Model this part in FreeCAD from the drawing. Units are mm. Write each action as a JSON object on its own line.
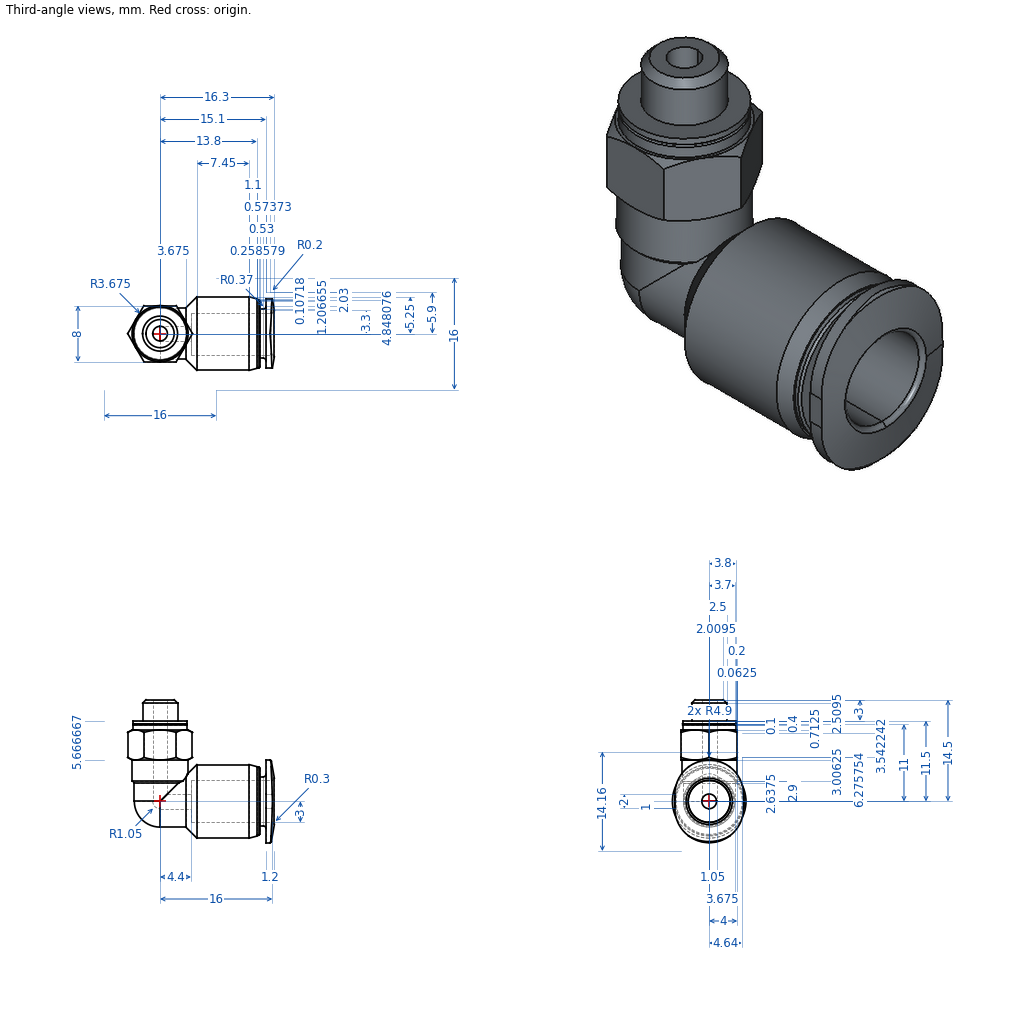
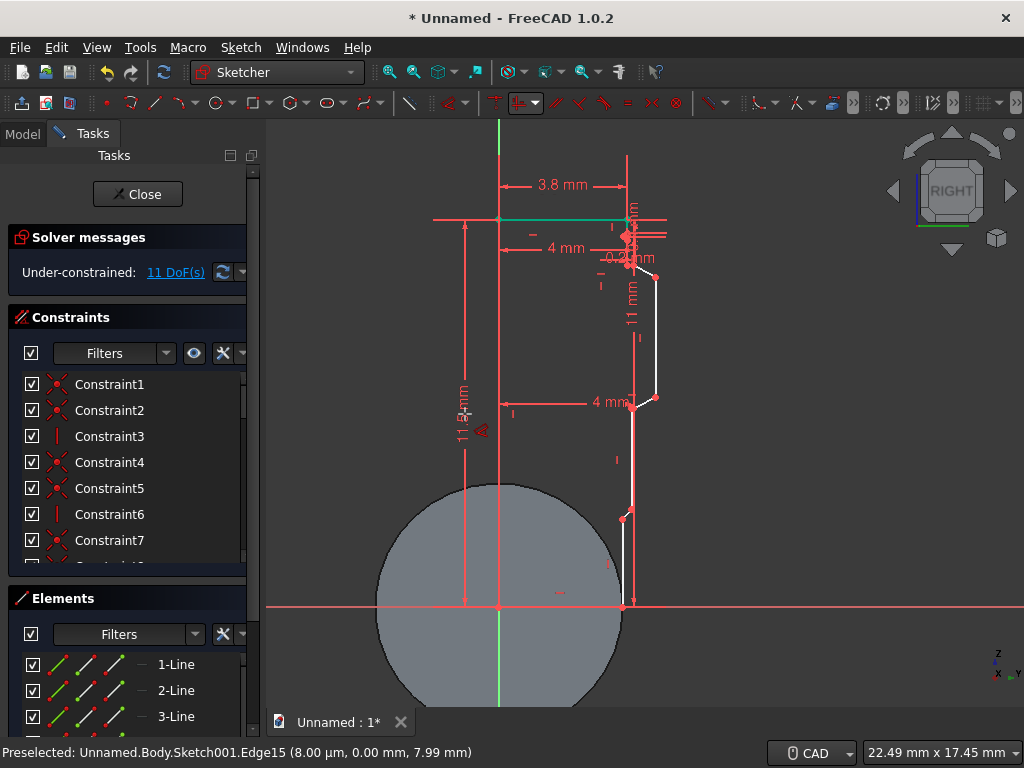
{"action": "left_click", "coordinate": [632, 510]}
{"action": "left_click", "coordinate": [465, 559]}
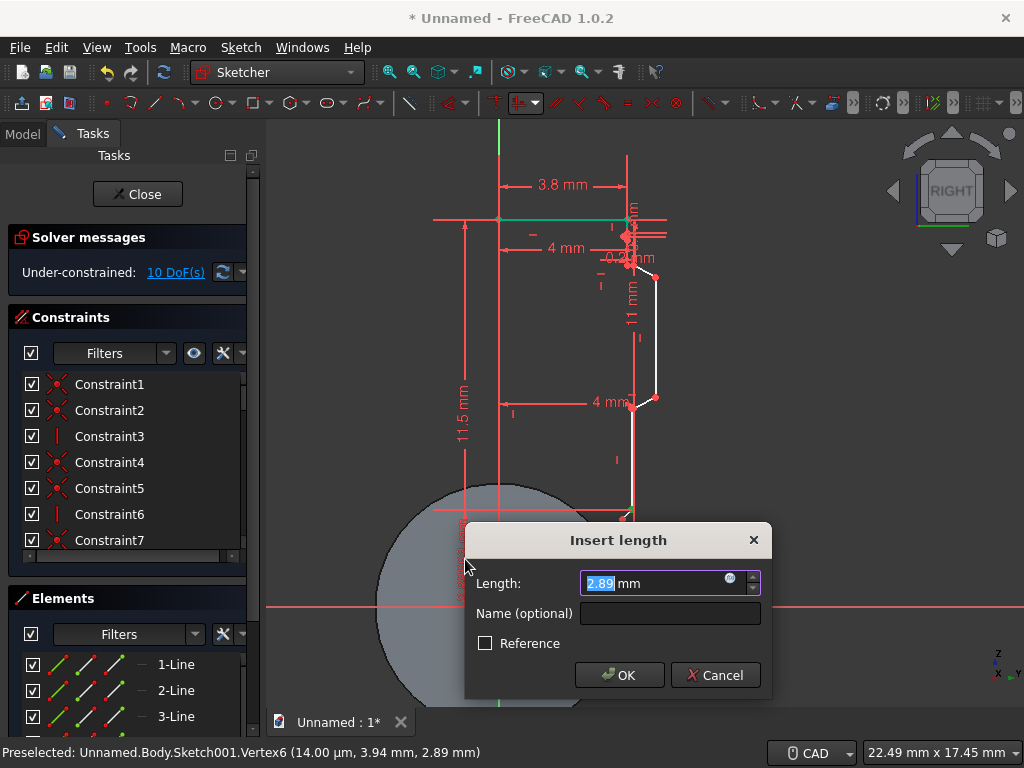
{"action": "type", "text": "2.9"}
{"action": "key", "text": "Return"}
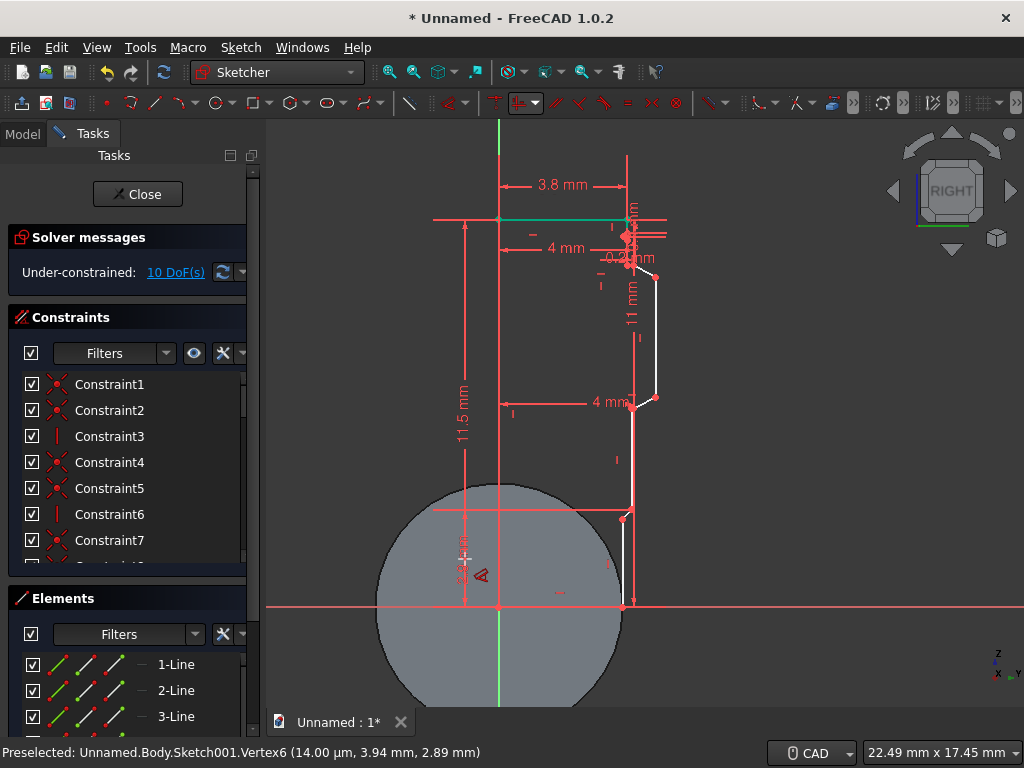
{"action": "scroll", "coordinate": [624, 237], "scroll_direction": "up", "scroll_amount": 5}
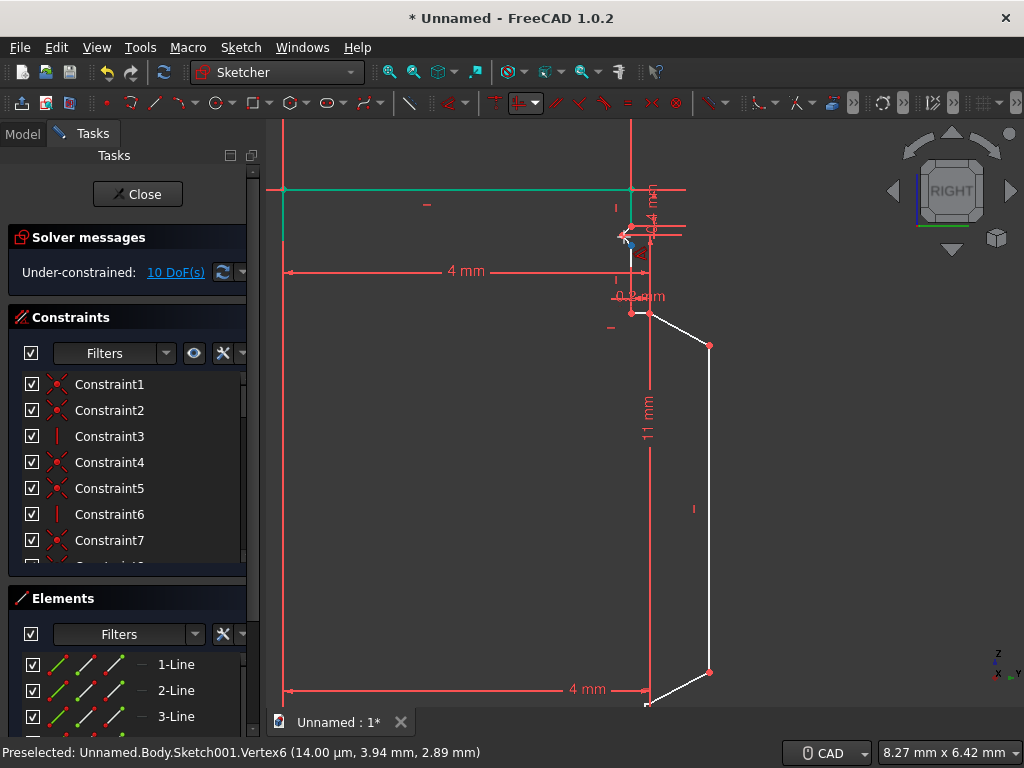
{"action": "left_click", "coordinate": [622, 235]}
{"action": "left_click", "coordinate": [458, 153]}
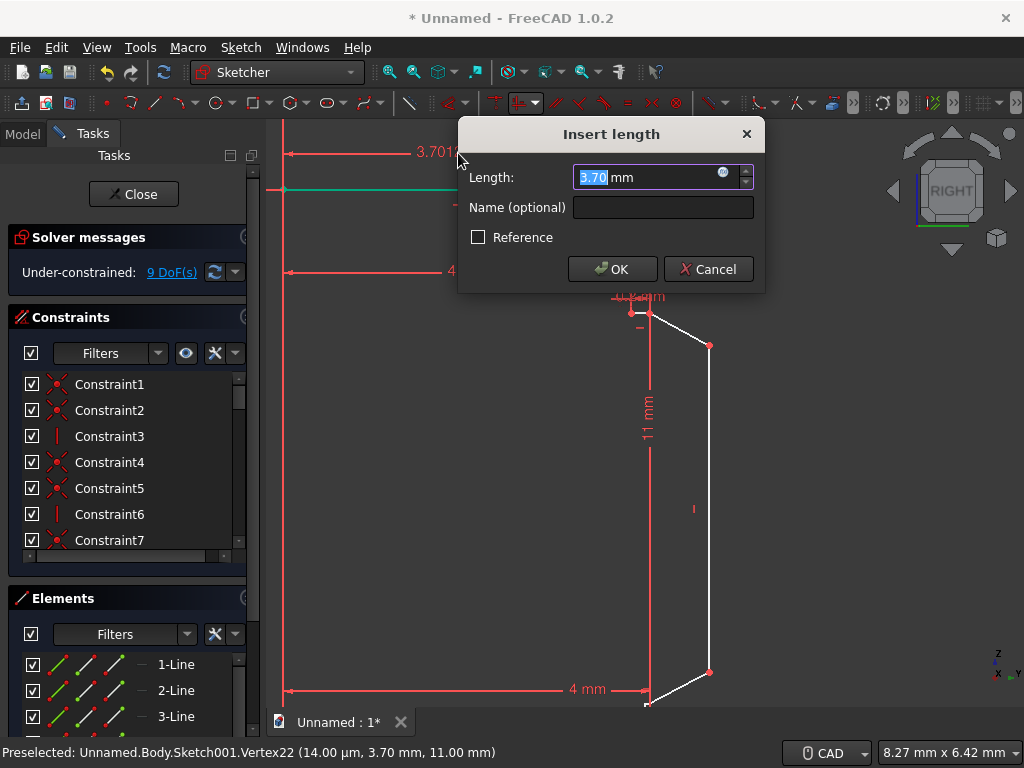
{"action": "type", "text": "3.7"}
{"action": "key", "text": "Return"}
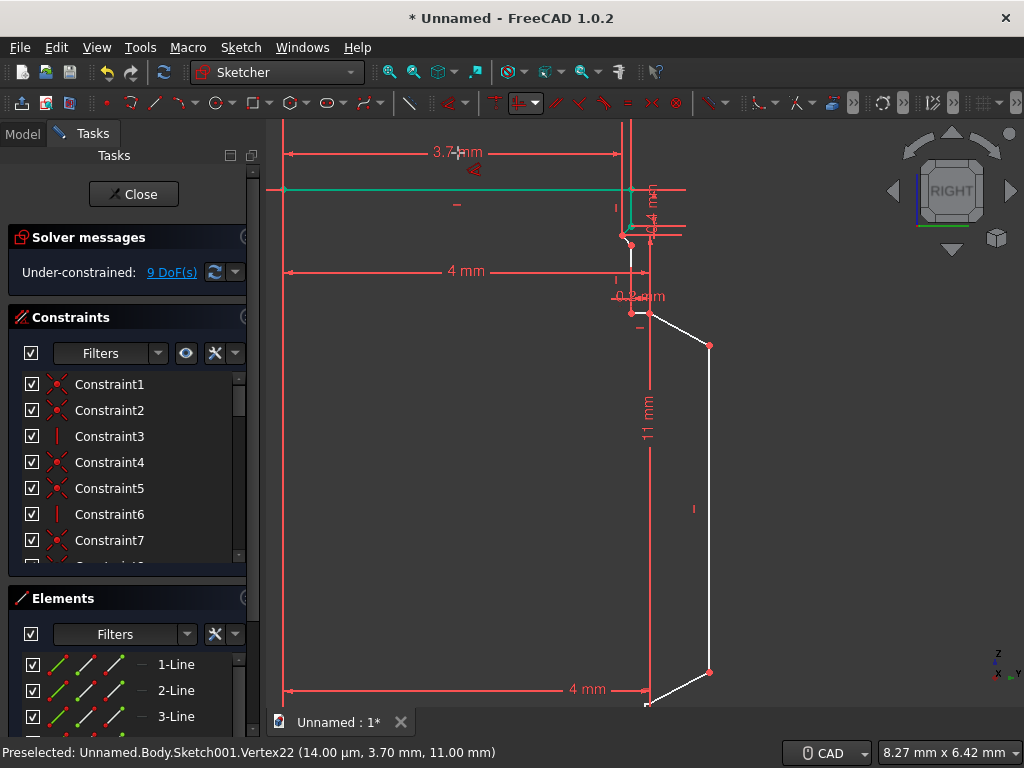
{"action": "scroll", "coordinate": [627, 241], "scroll_direction": "up", "scroll_amount": 8}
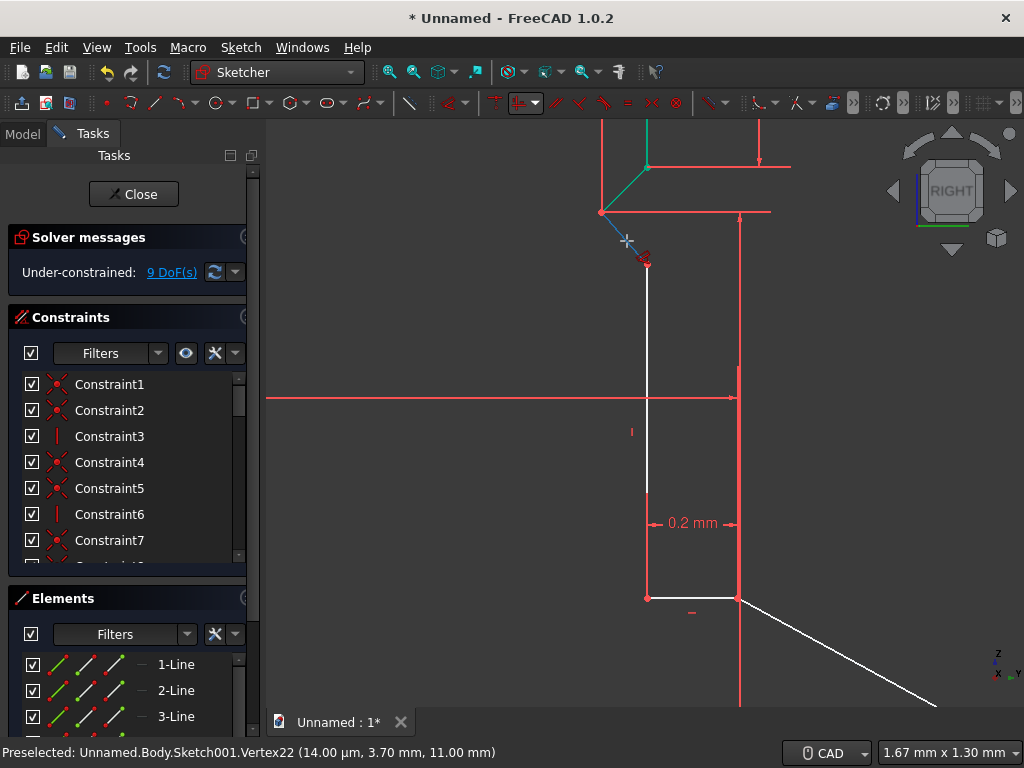
{"action": "left_click", "coordinate": [624, 239]}
{"action": "left_click", "coordinate": [681, 239]}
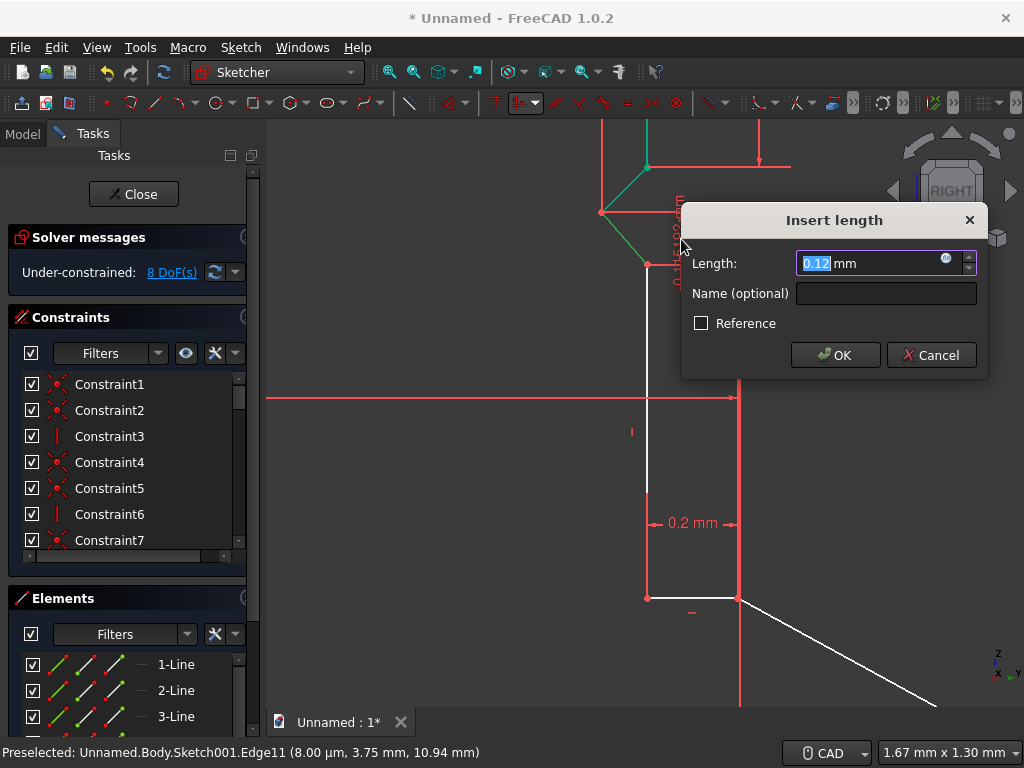
{"action": "type", "text": "0.1"}
{"action": "key", "text": "Return"}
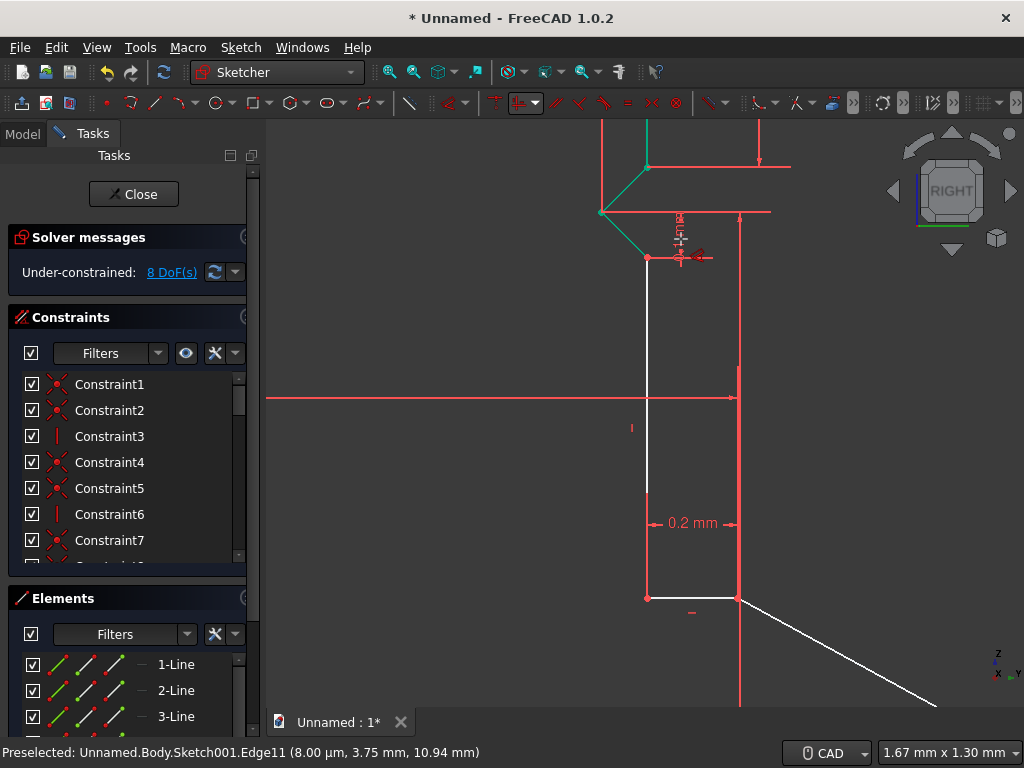
{"action": "scroll", "coordinate": [625, 238], "scroll_direction": "down", "scroll_amount": 13}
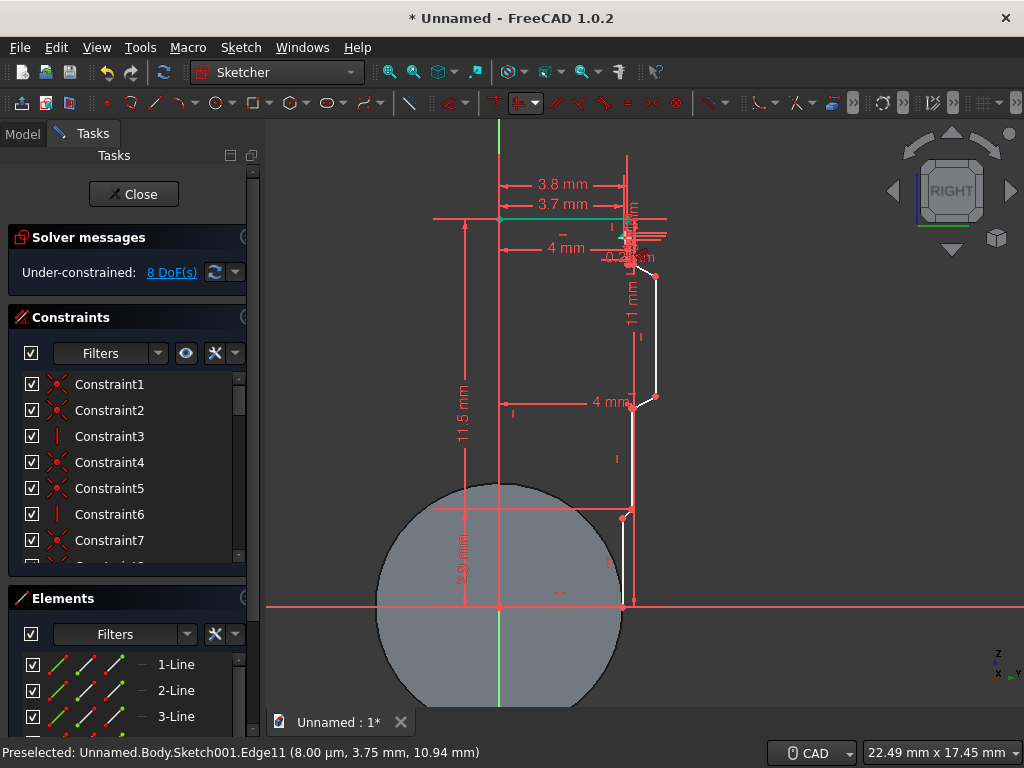
{"action": "left_click", "coordinate": [536, 607]}
{"action": "left_click", "coordinate": [561, 641]}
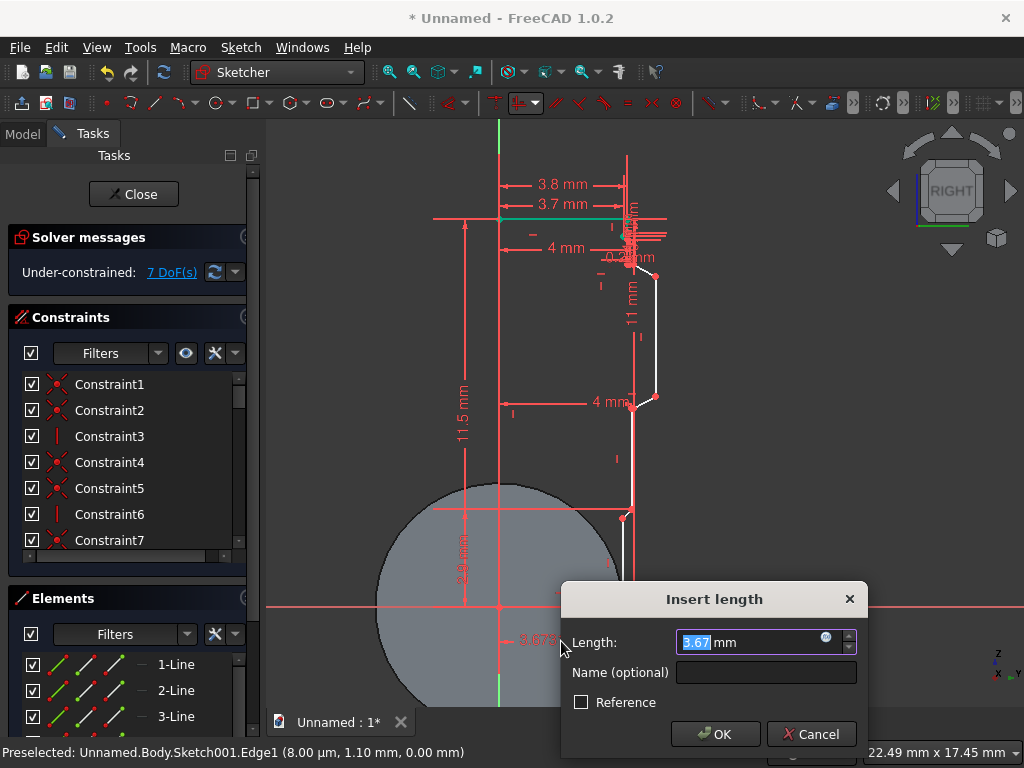
{"action": "type", "text": "3.675"}
{"action": "key", "text": "Return"}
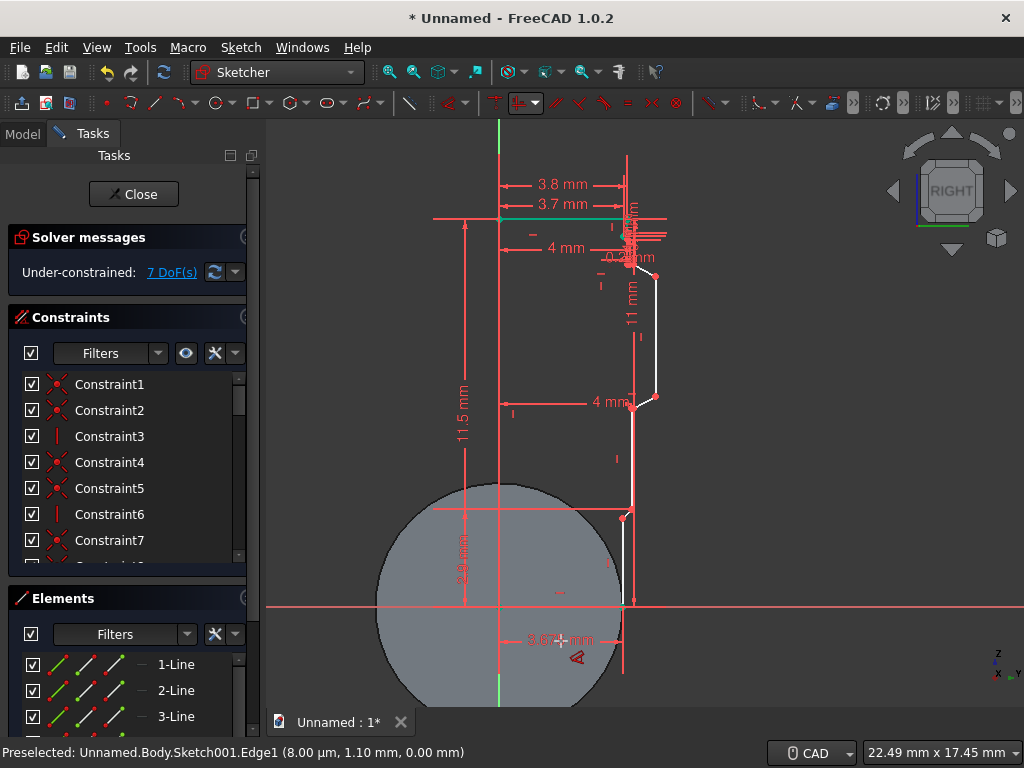
{"action": "left_click", "coordinate": [656, 397]}
{"action": "left_click", "coordinate": [632, 641]}